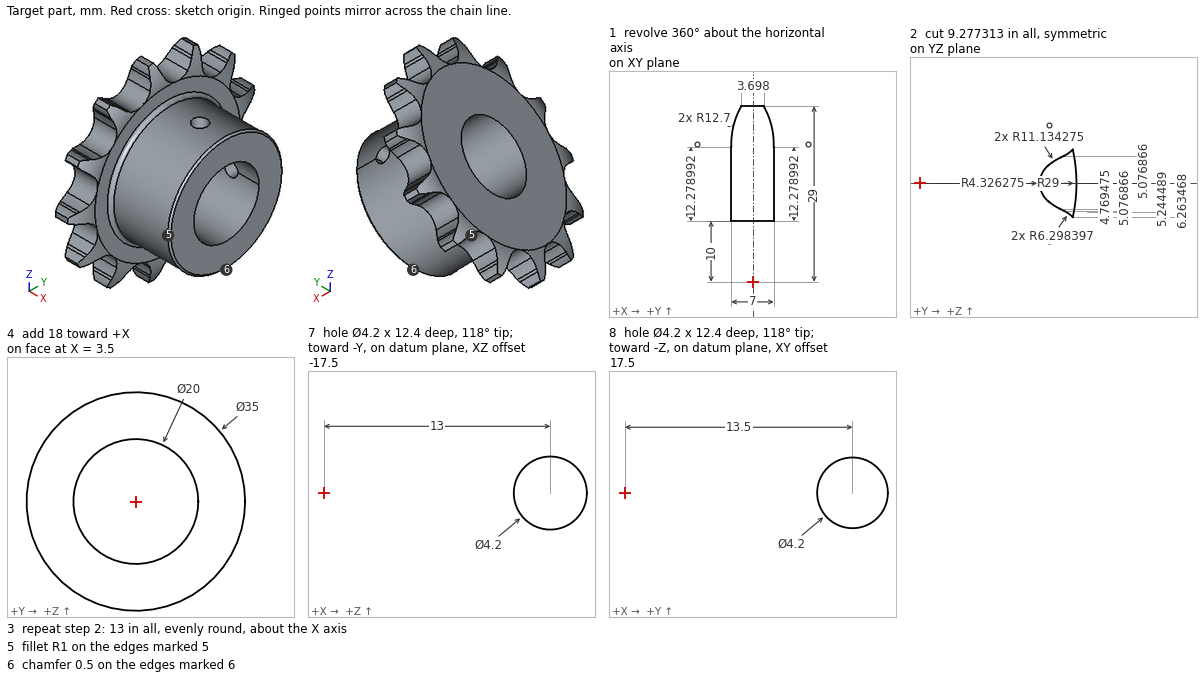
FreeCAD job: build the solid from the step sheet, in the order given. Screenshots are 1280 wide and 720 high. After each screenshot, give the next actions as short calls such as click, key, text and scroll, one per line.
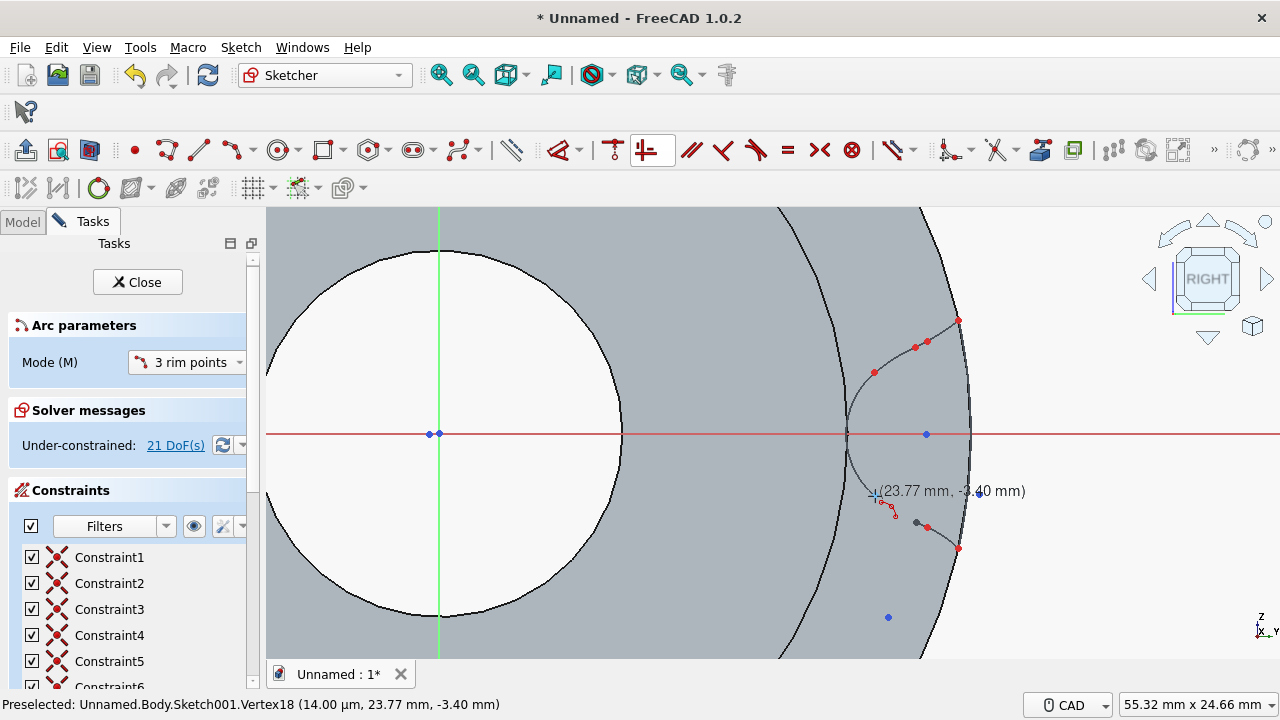
scroll(916, 521, up, 5)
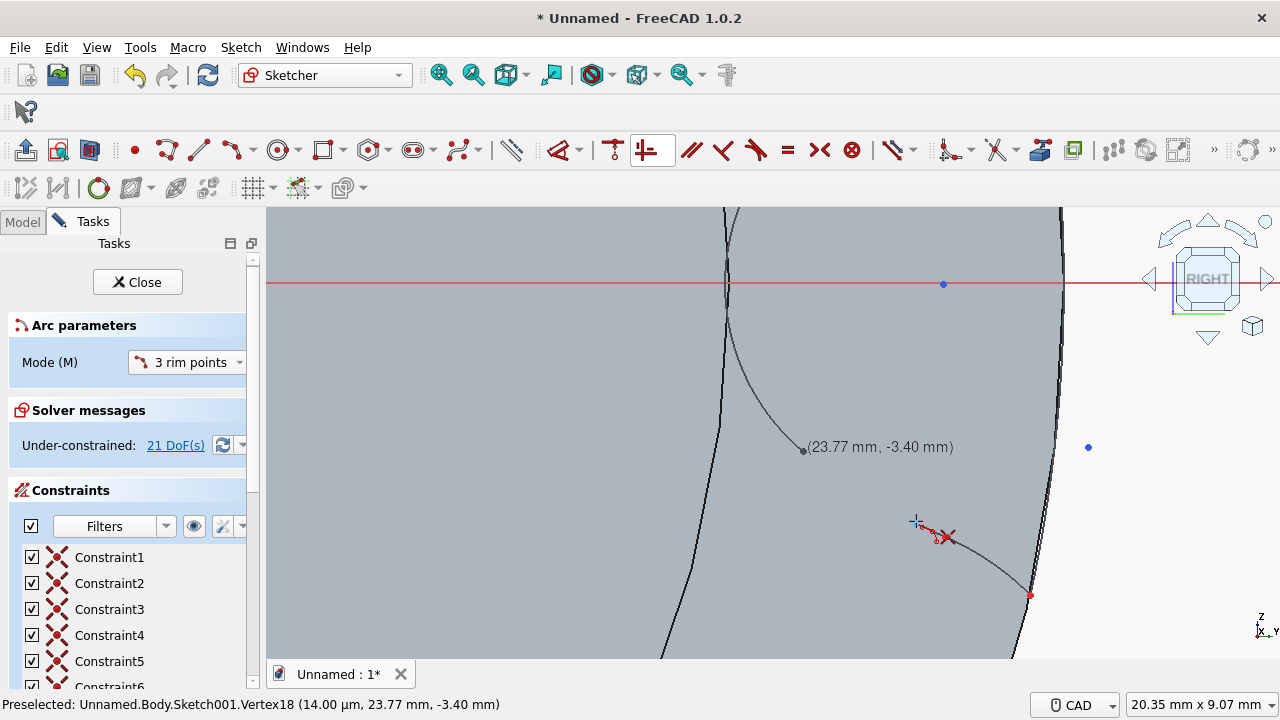
click(915, 523)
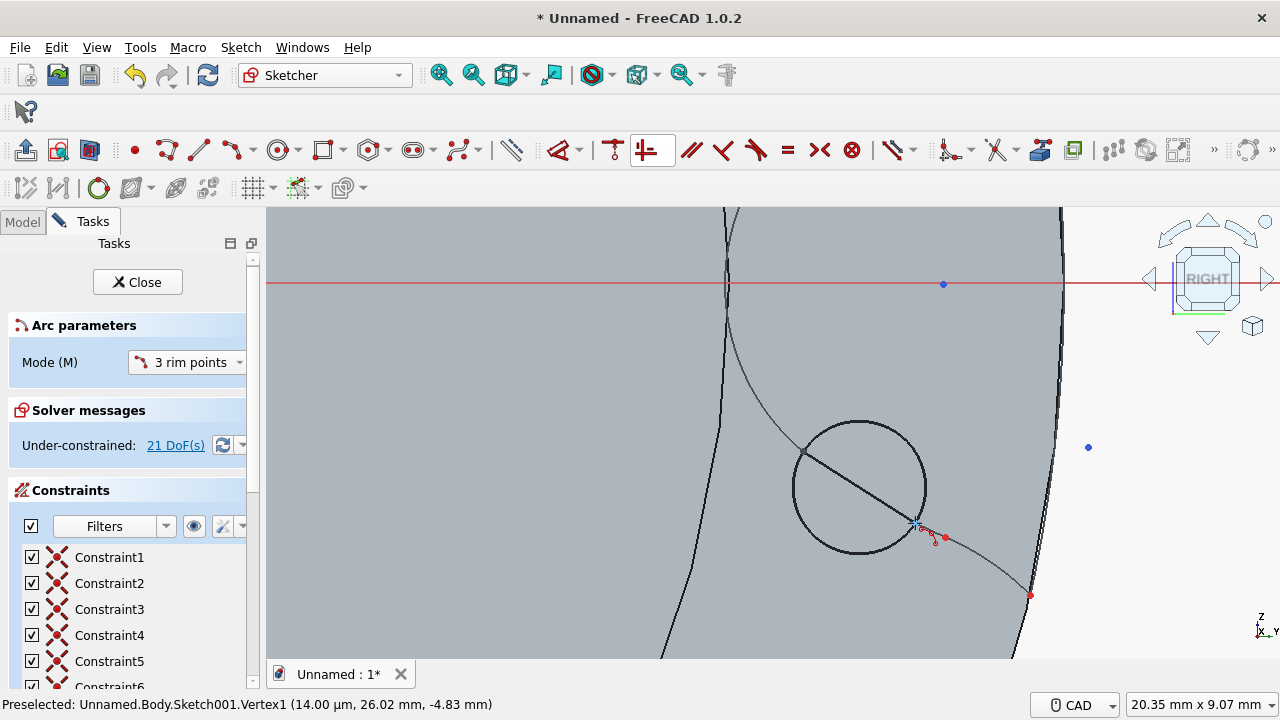
scroll(857, 488, up, 7)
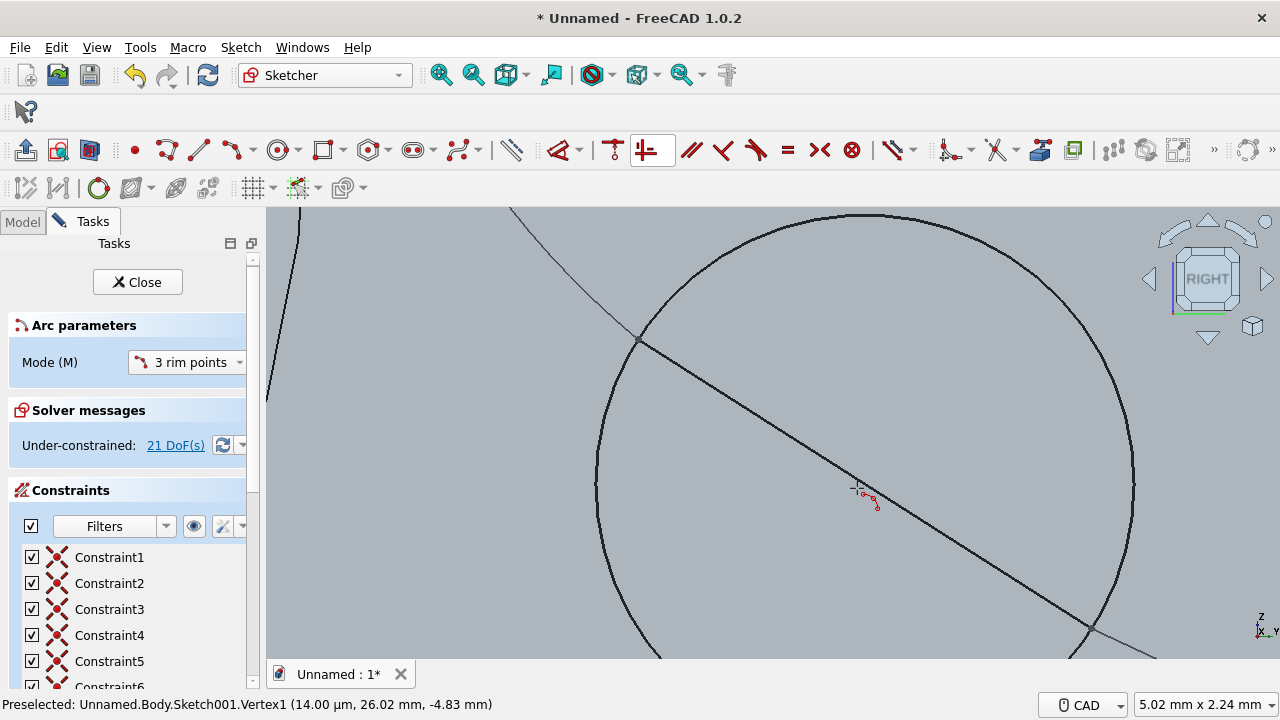
click(856, 485)
key(Escape)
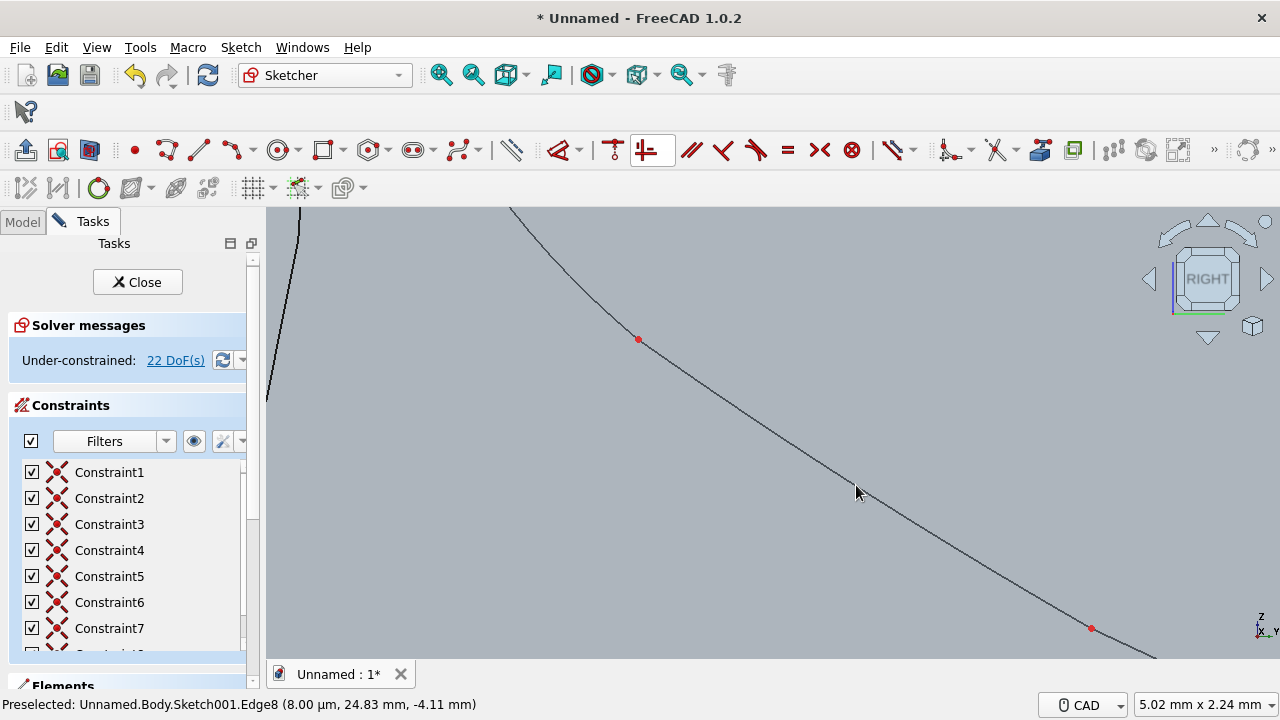
scroll(898, 511, down, 12)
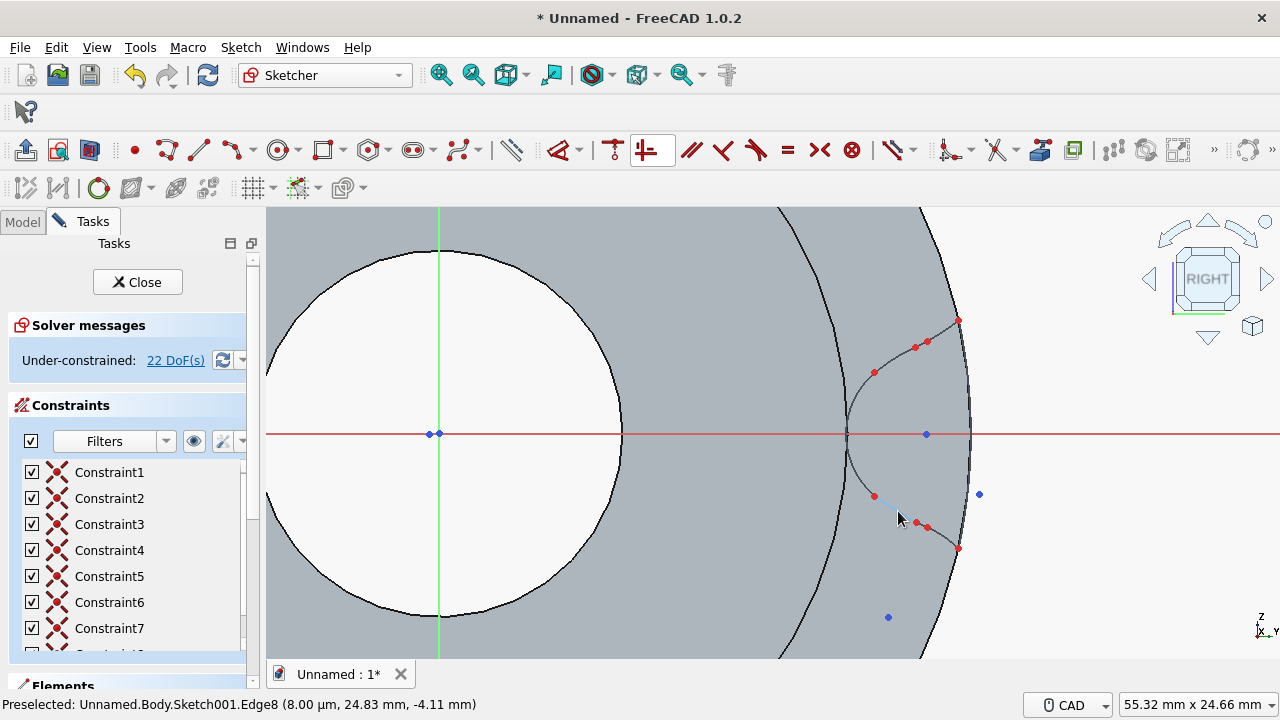
scroll(920, 524, up, 7)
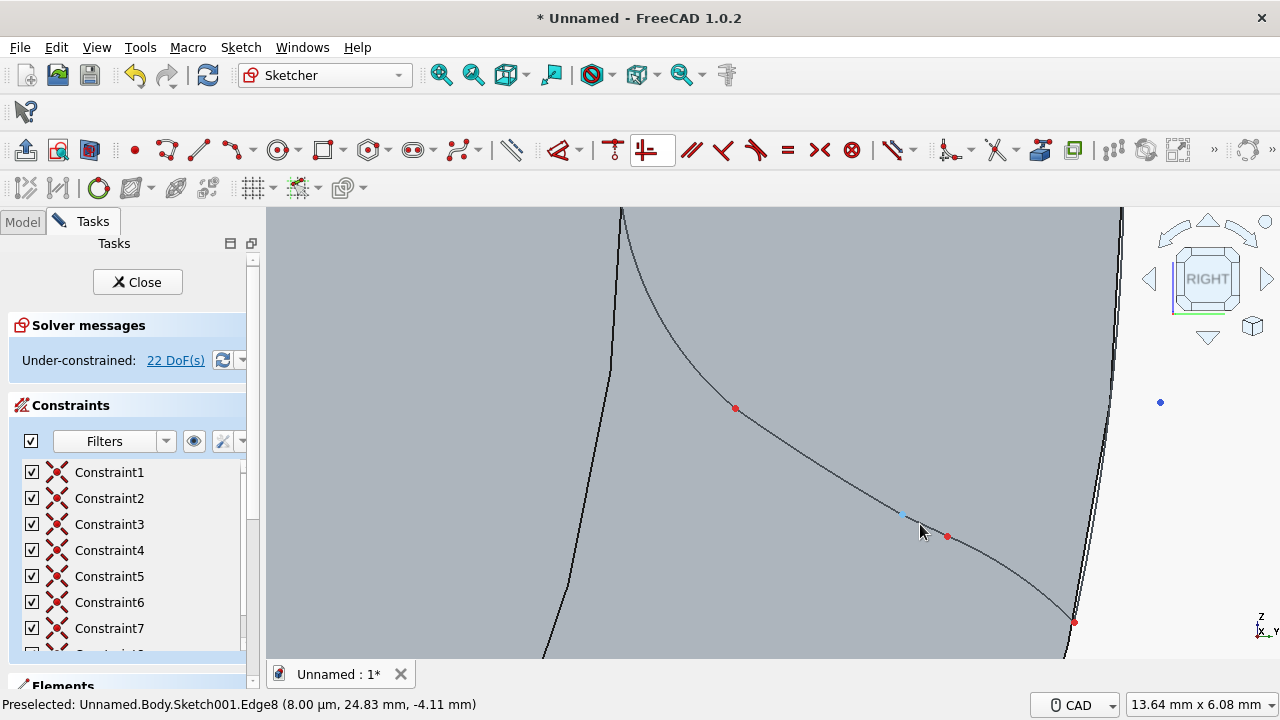
click(916, 521)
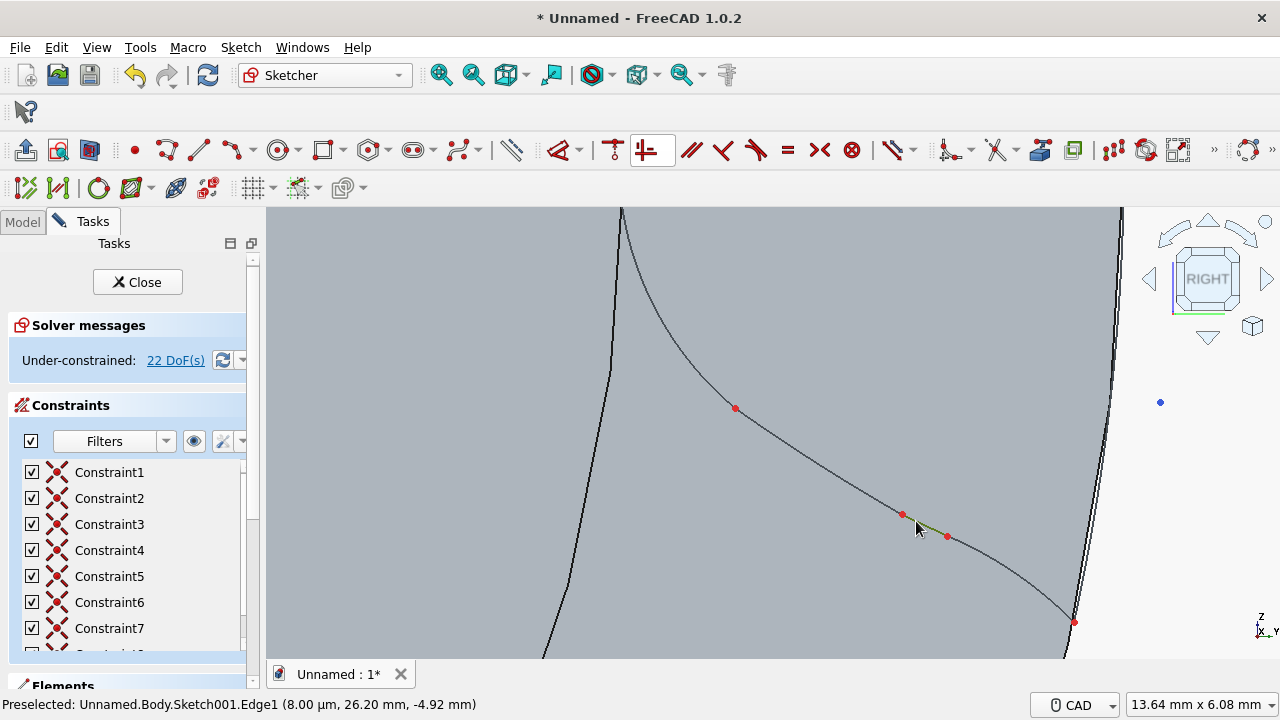
scroll(920, 524, down, 7)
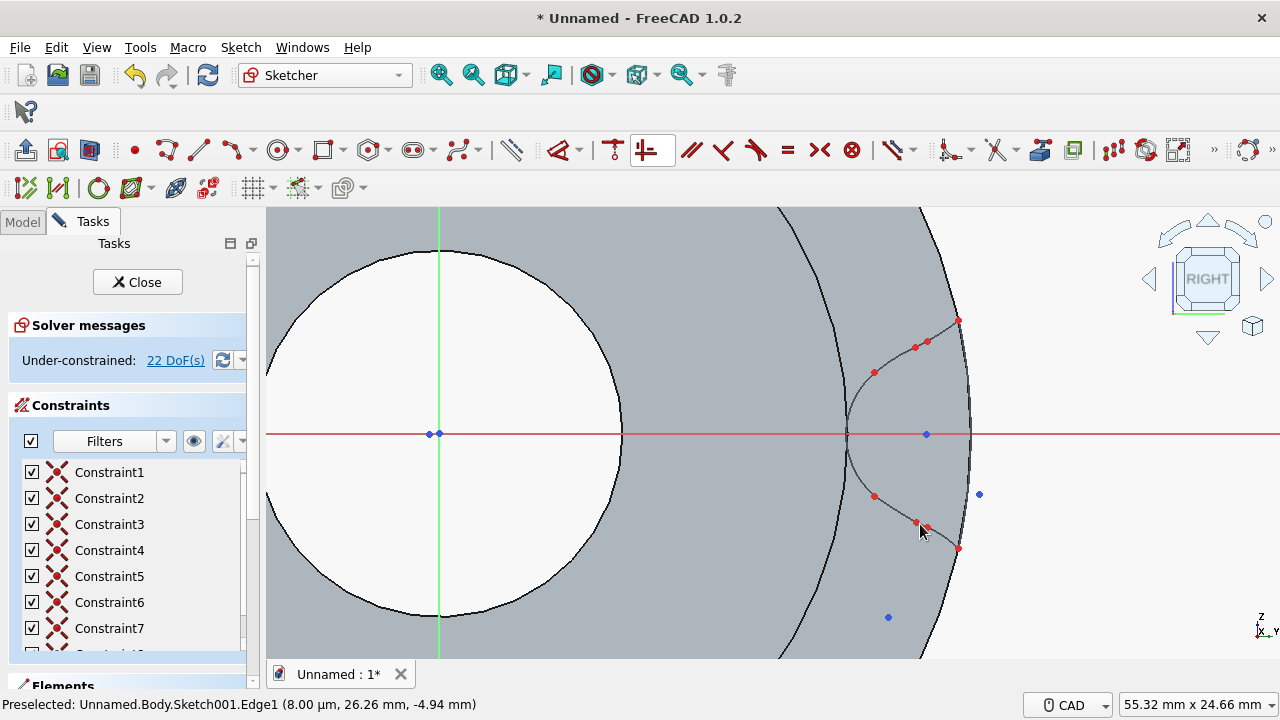
scroll(950, 541, up, 2)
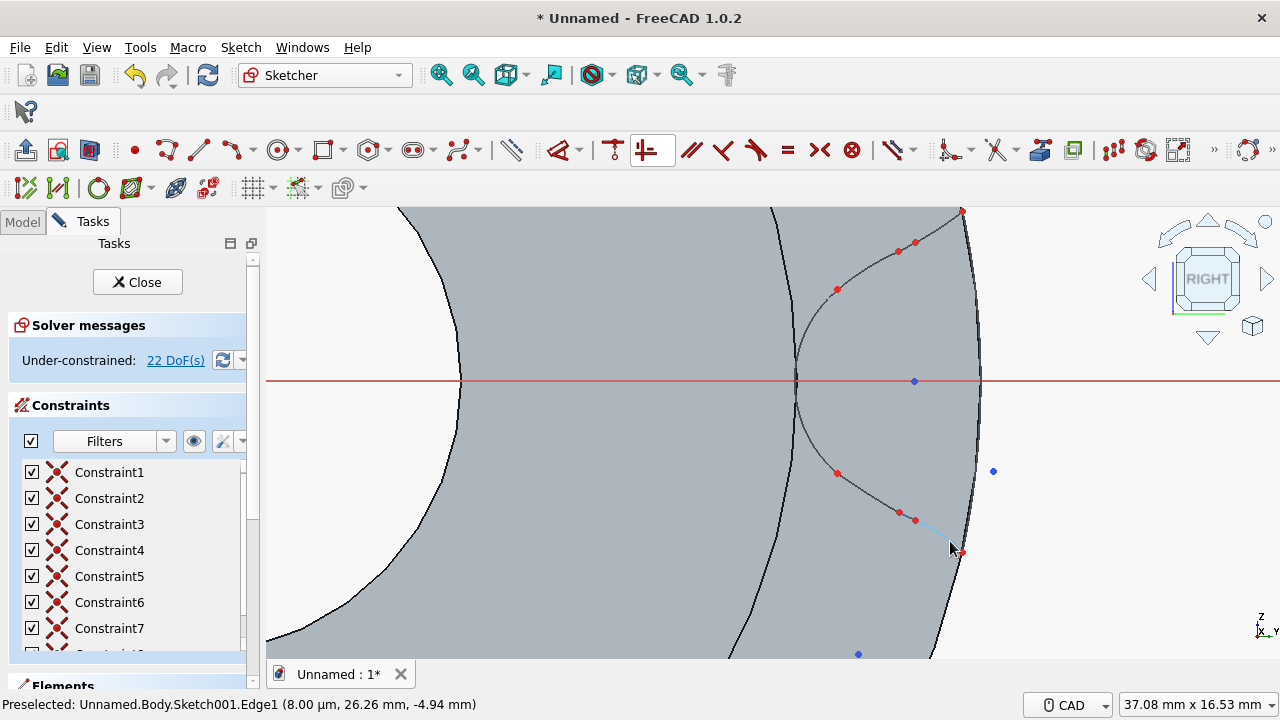
click(950, 541)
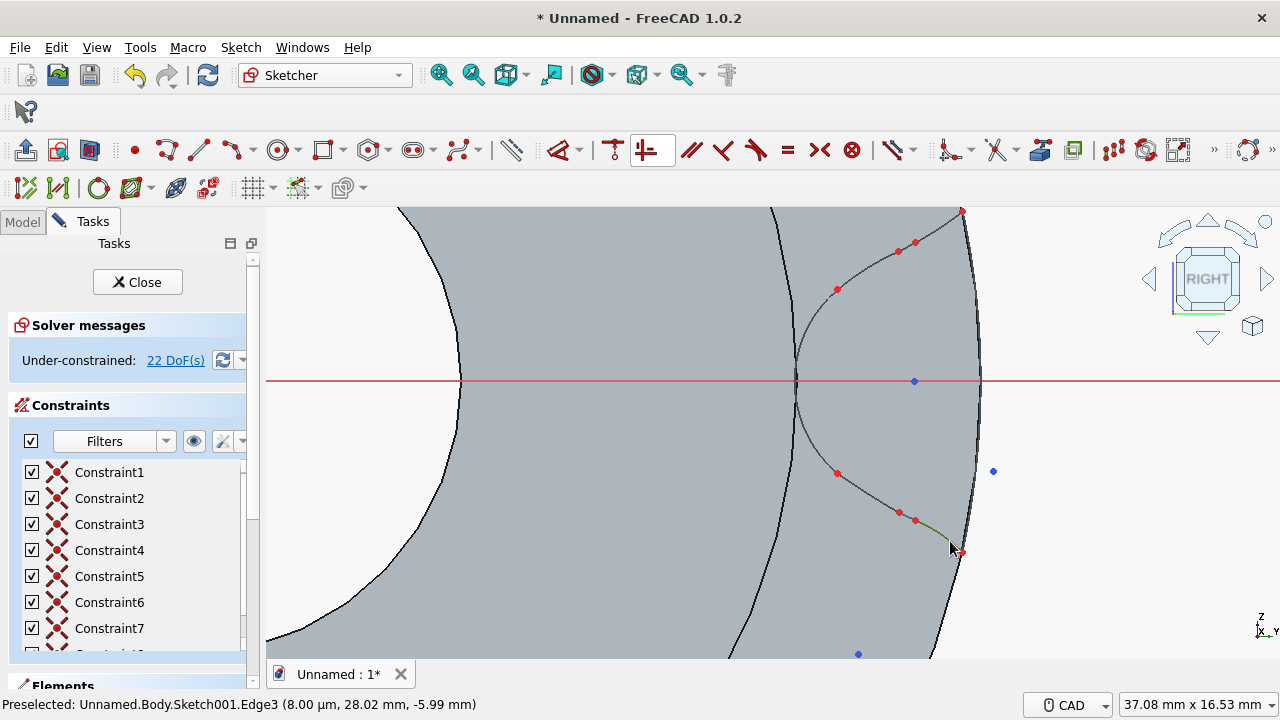
click(756, 150)